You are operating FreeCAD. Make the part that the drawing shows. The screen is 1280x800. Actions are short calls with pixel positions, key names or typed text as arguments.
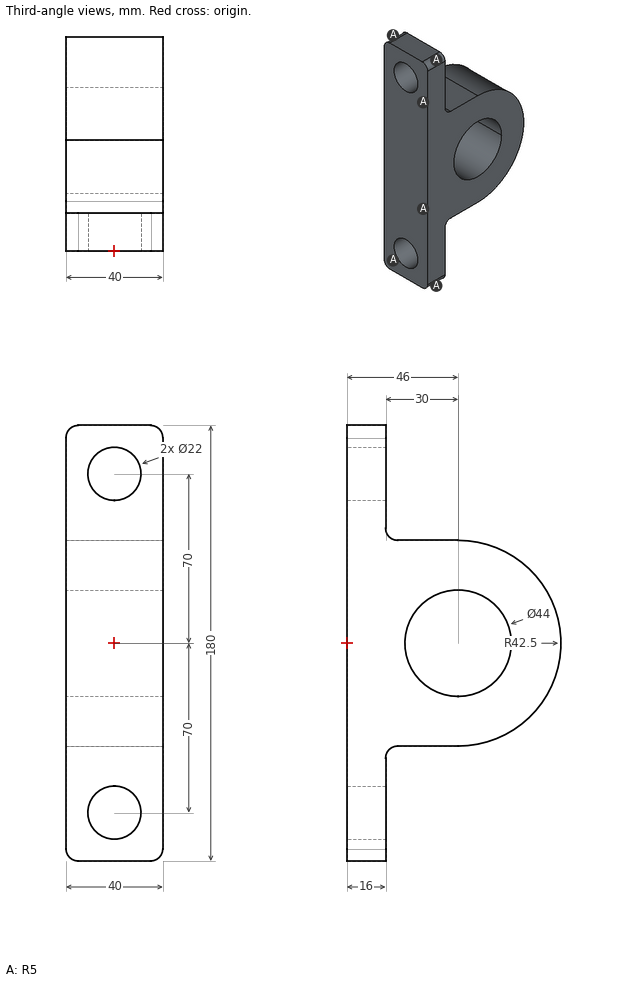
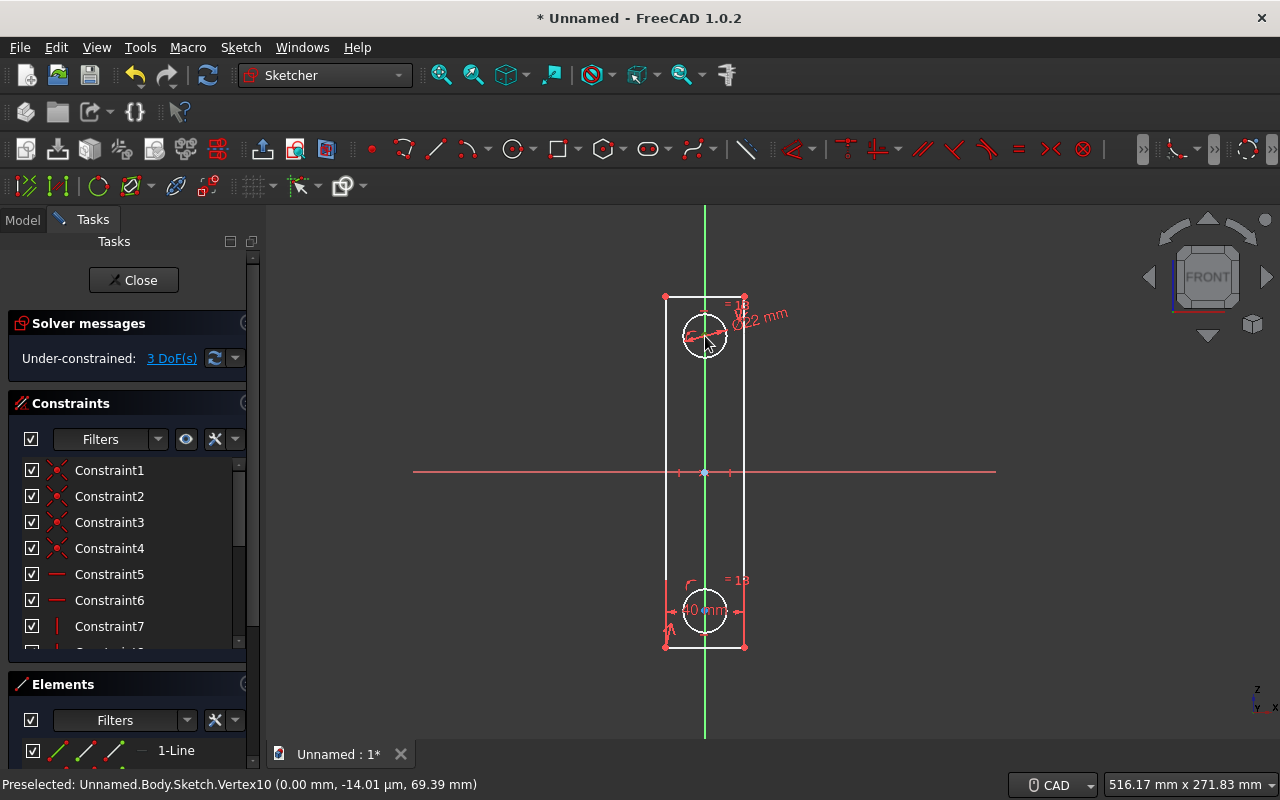
key(i)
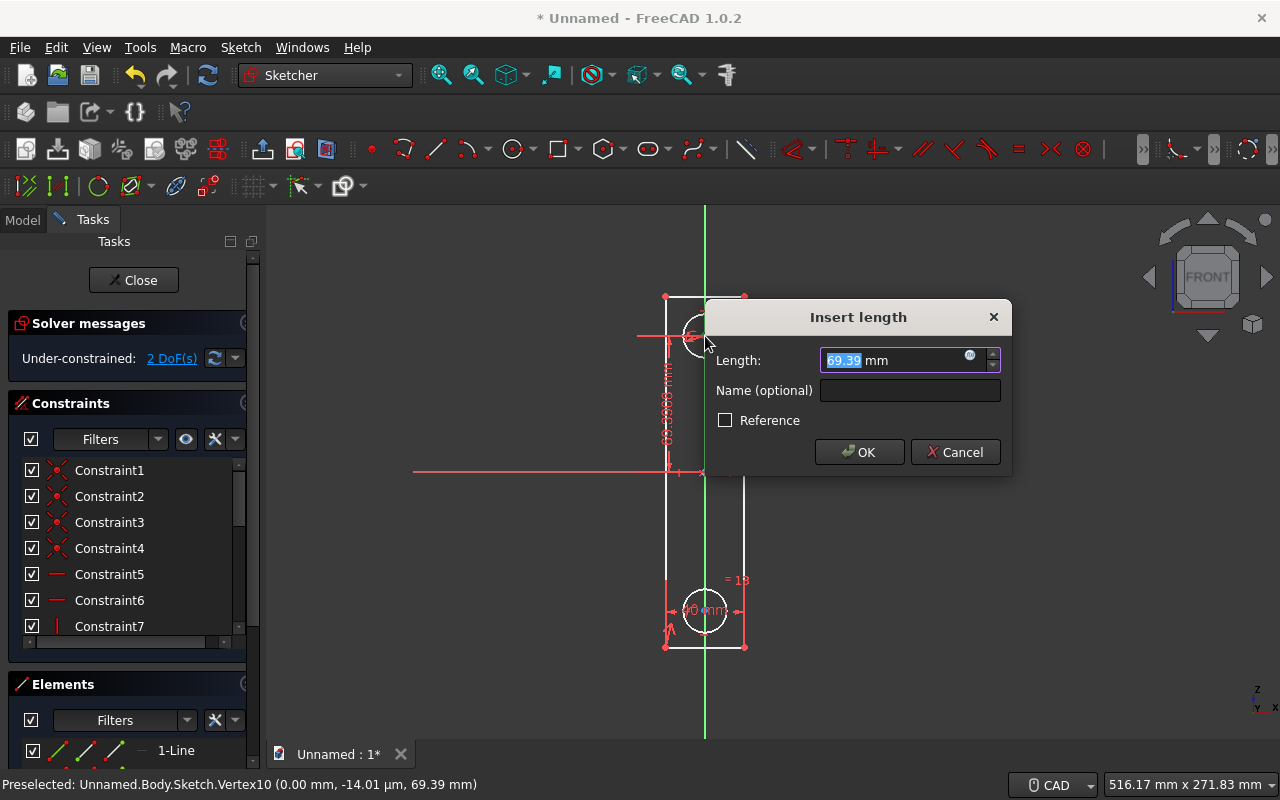
text(70)
key(Return)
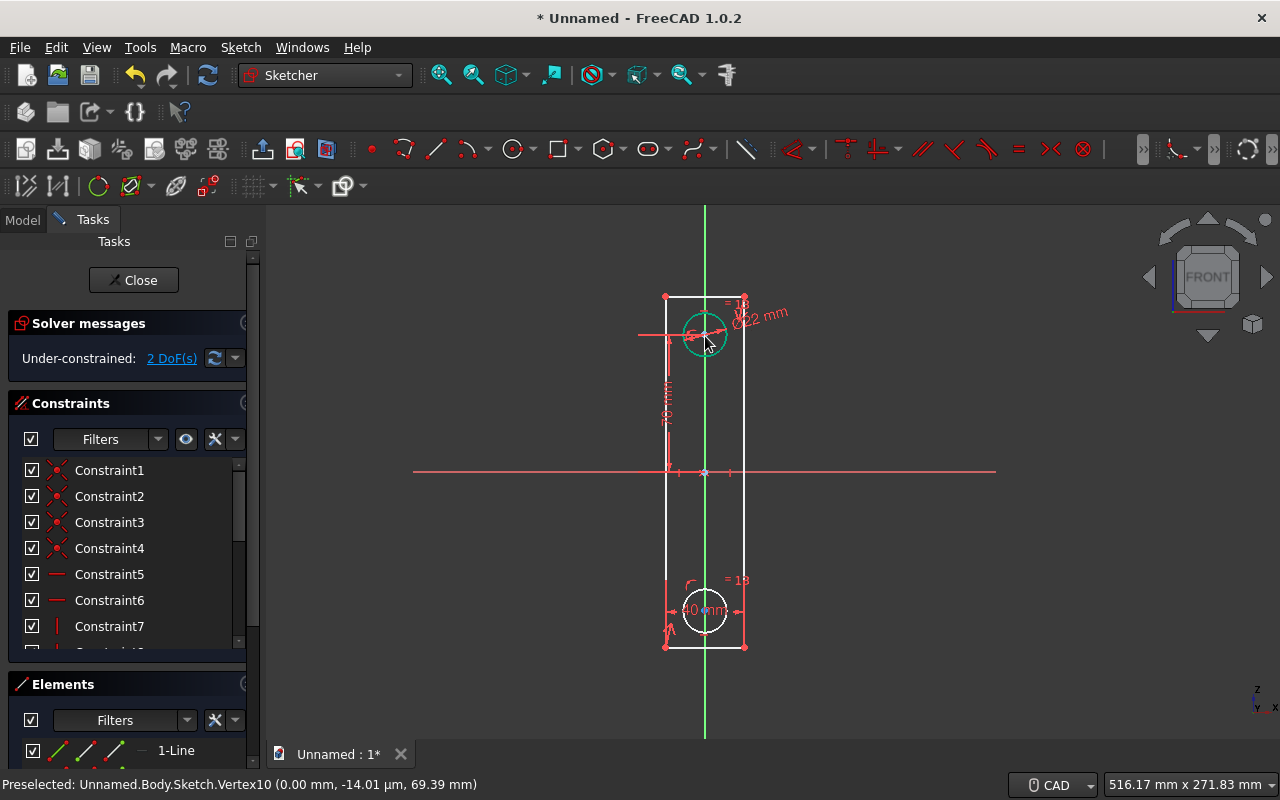
click(705, 611)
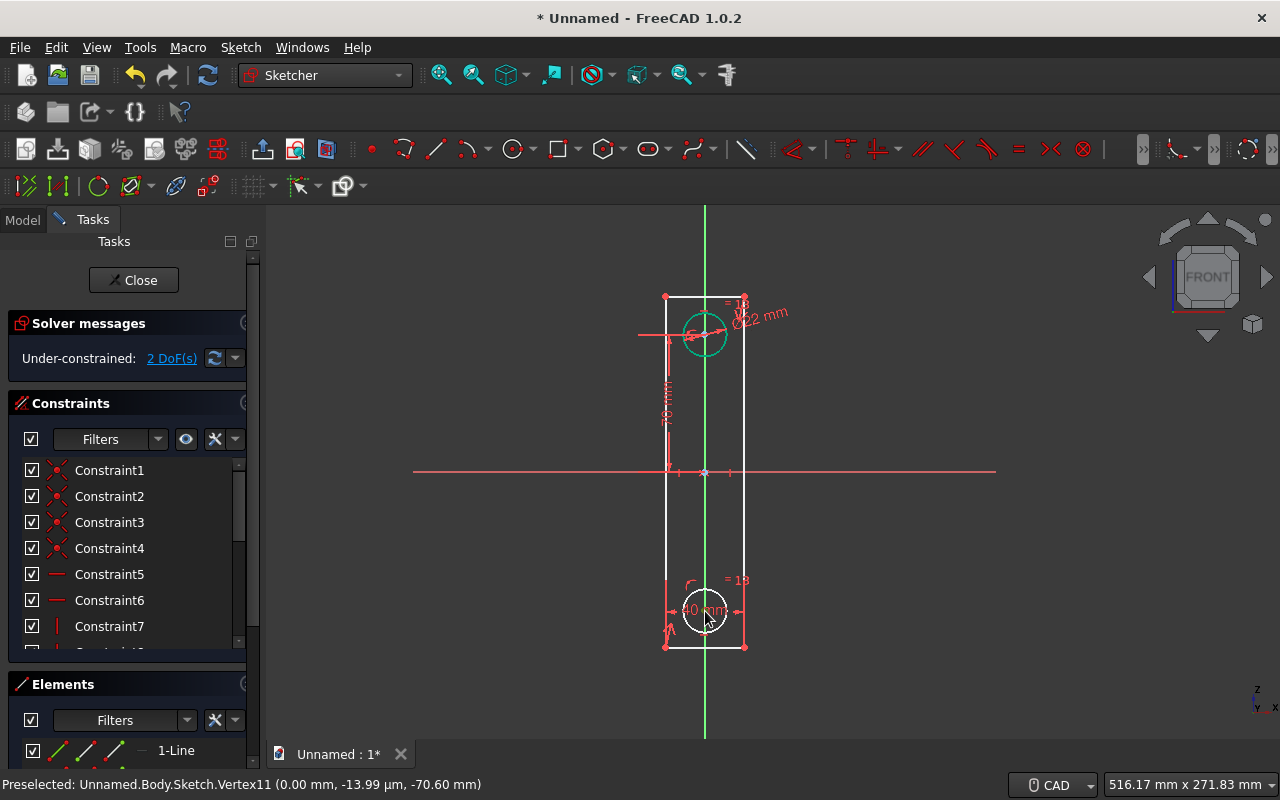
key(i)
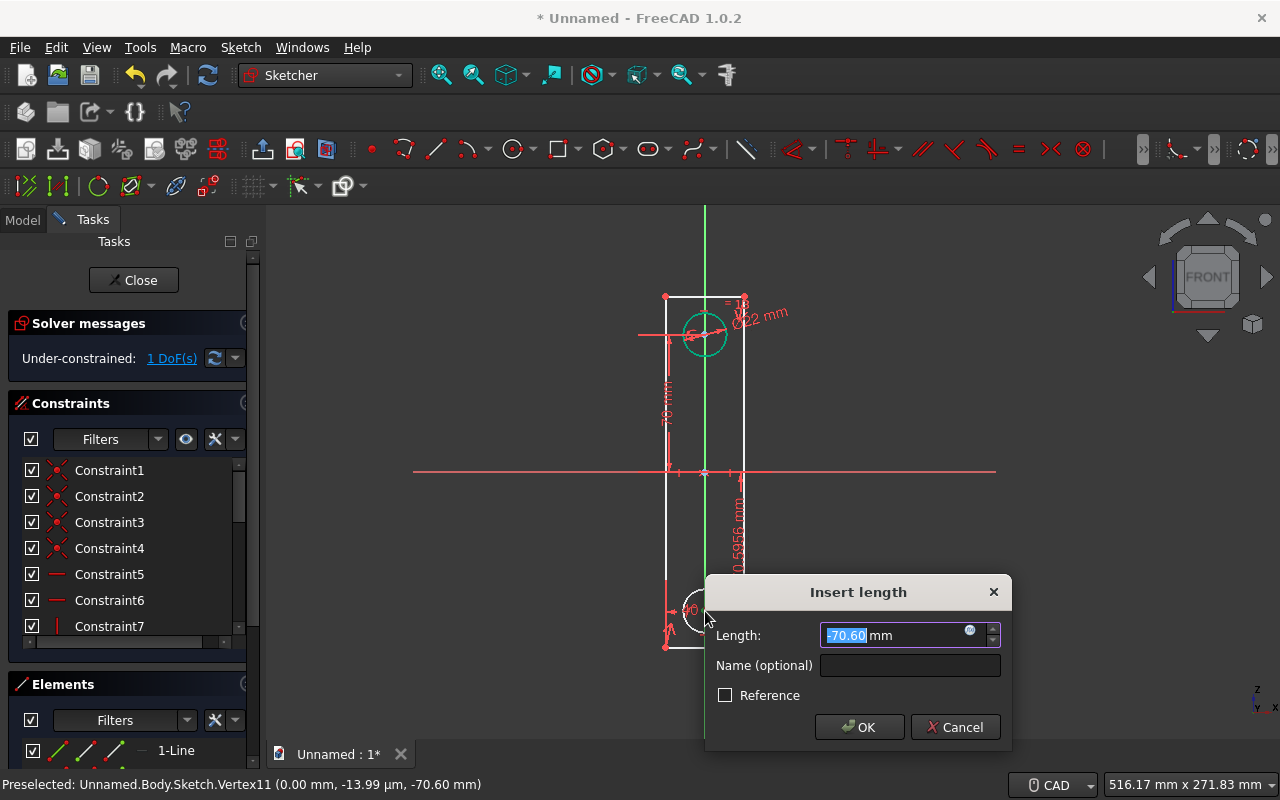
text(-70)
key(Return)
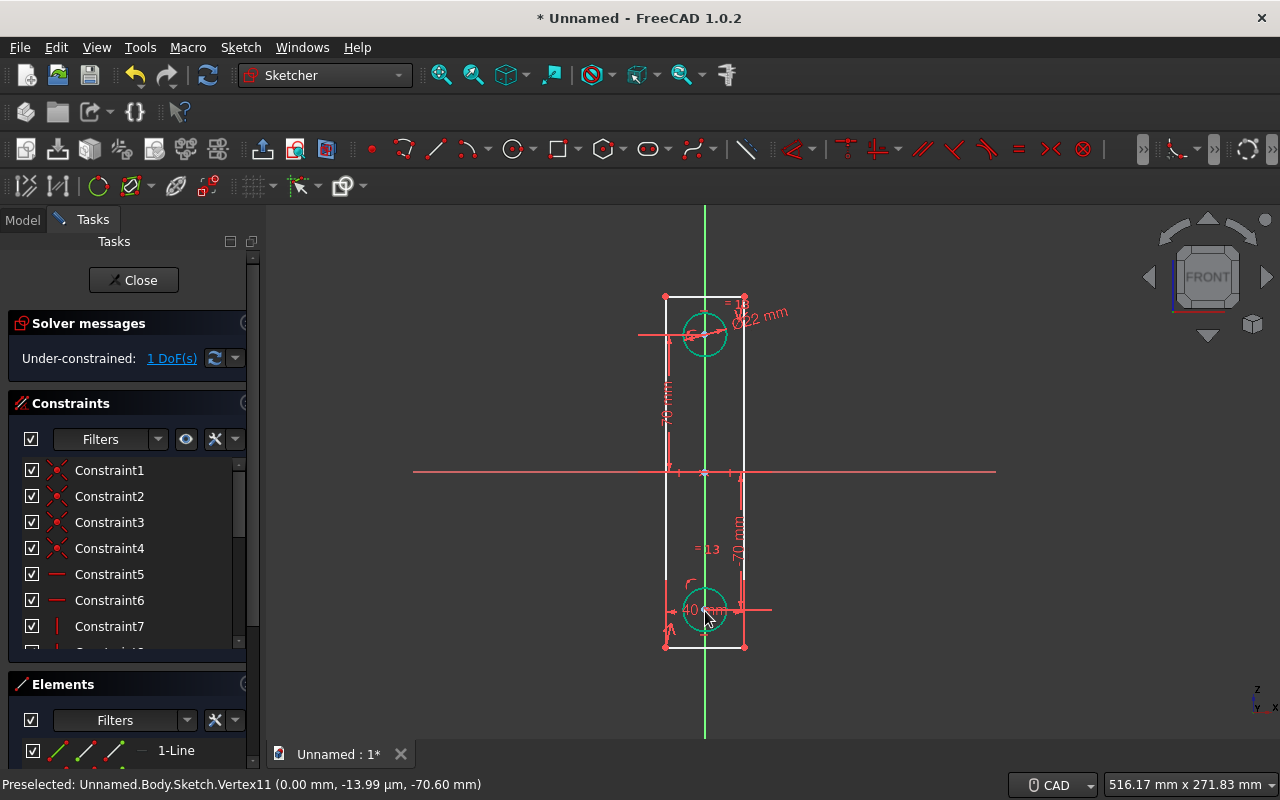
click(744, 402)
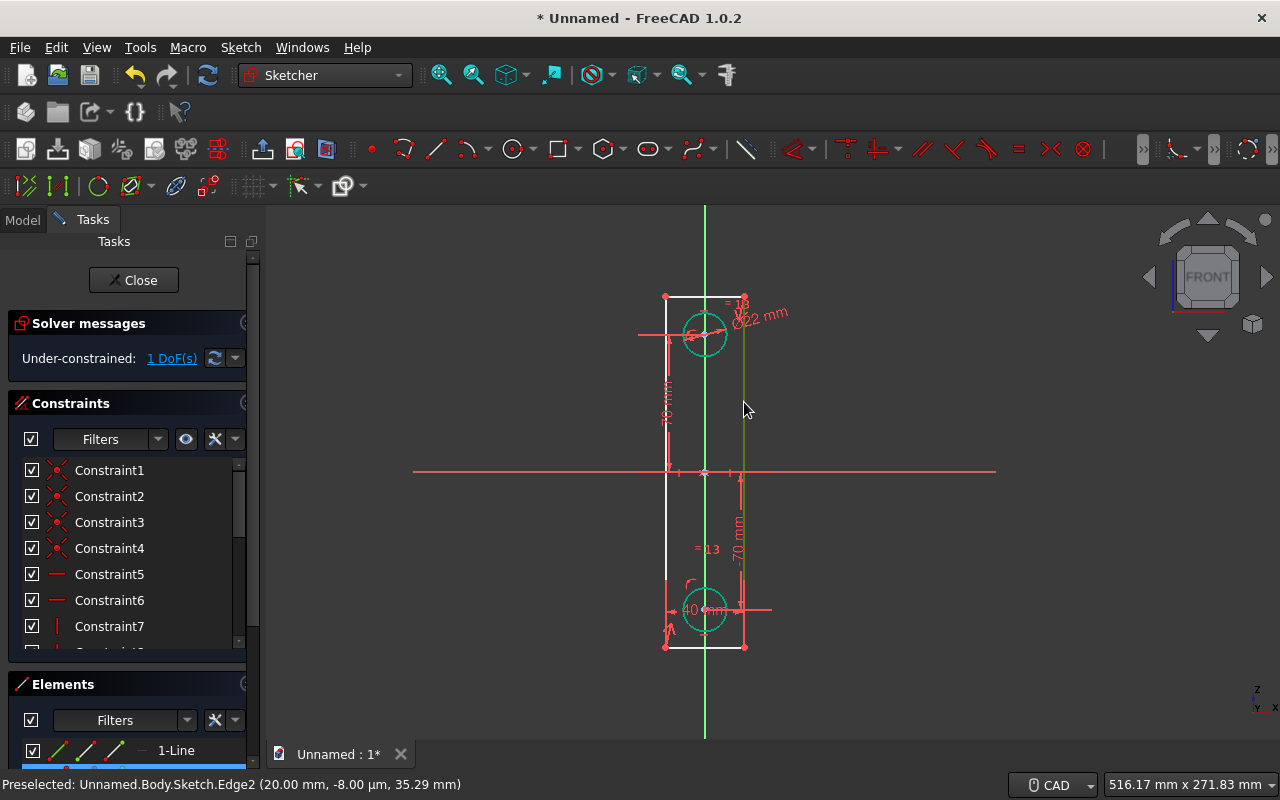
key(i)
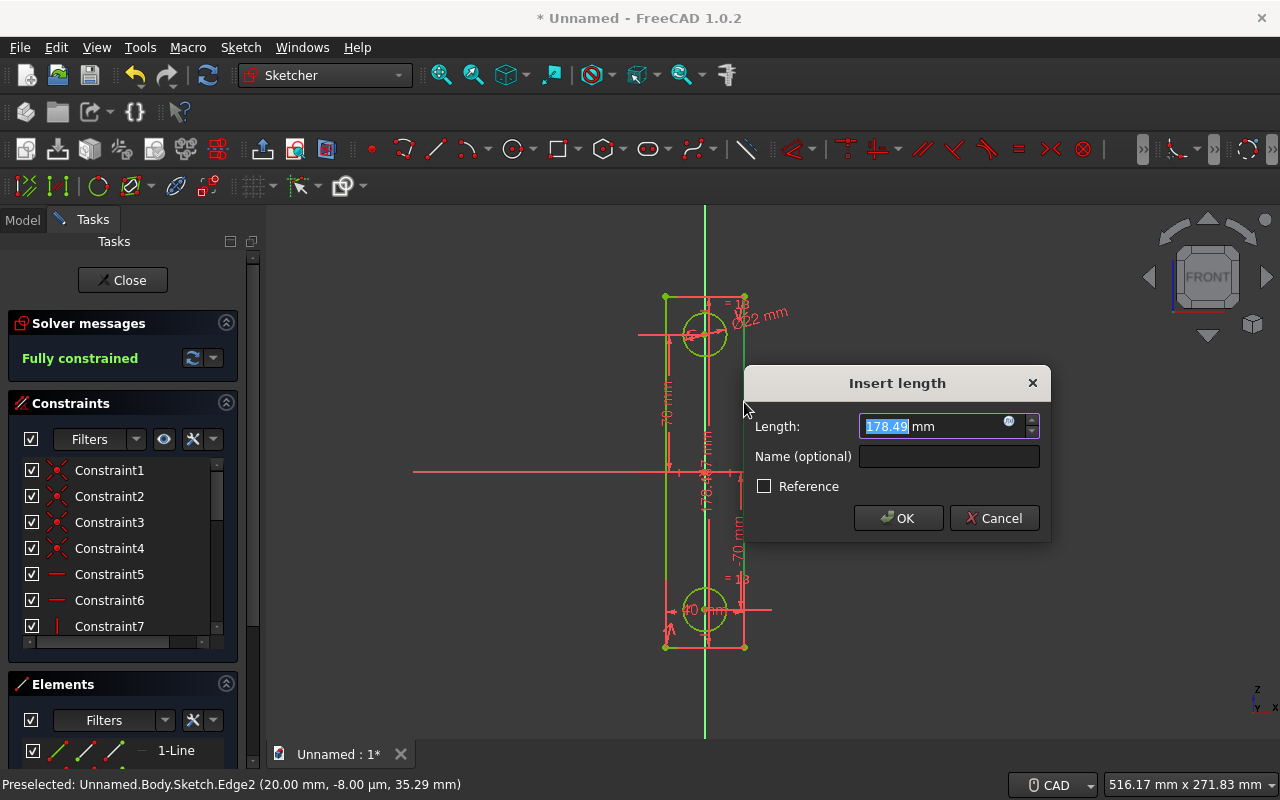
text(180)
key(Return)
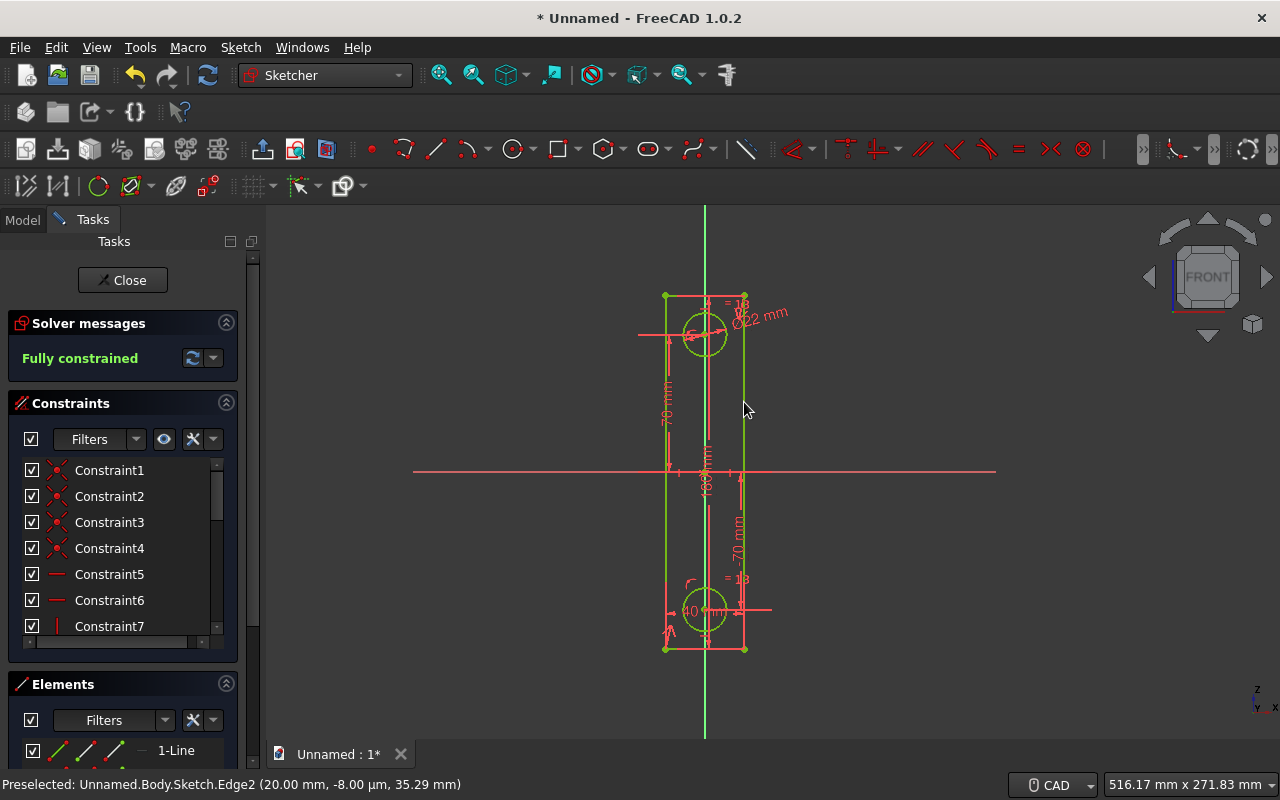
click(123, 280)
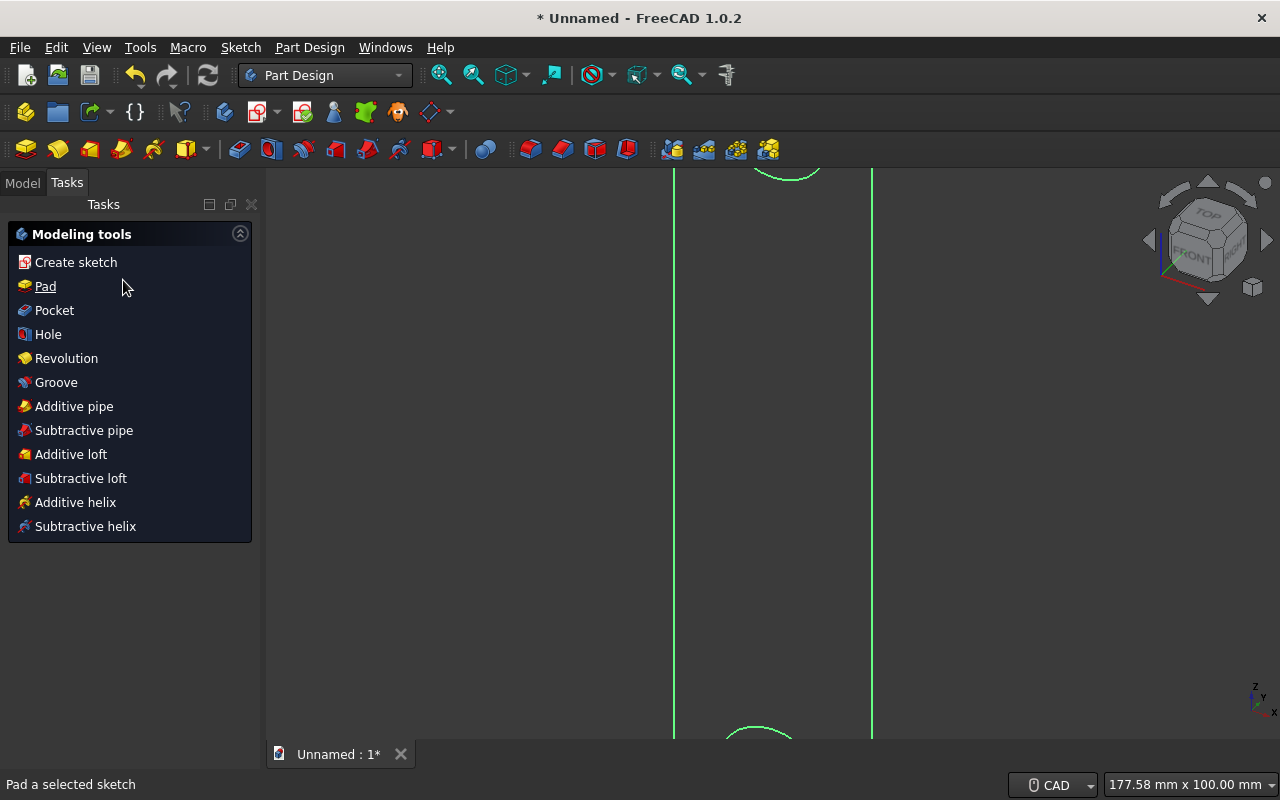
click(26, 150)